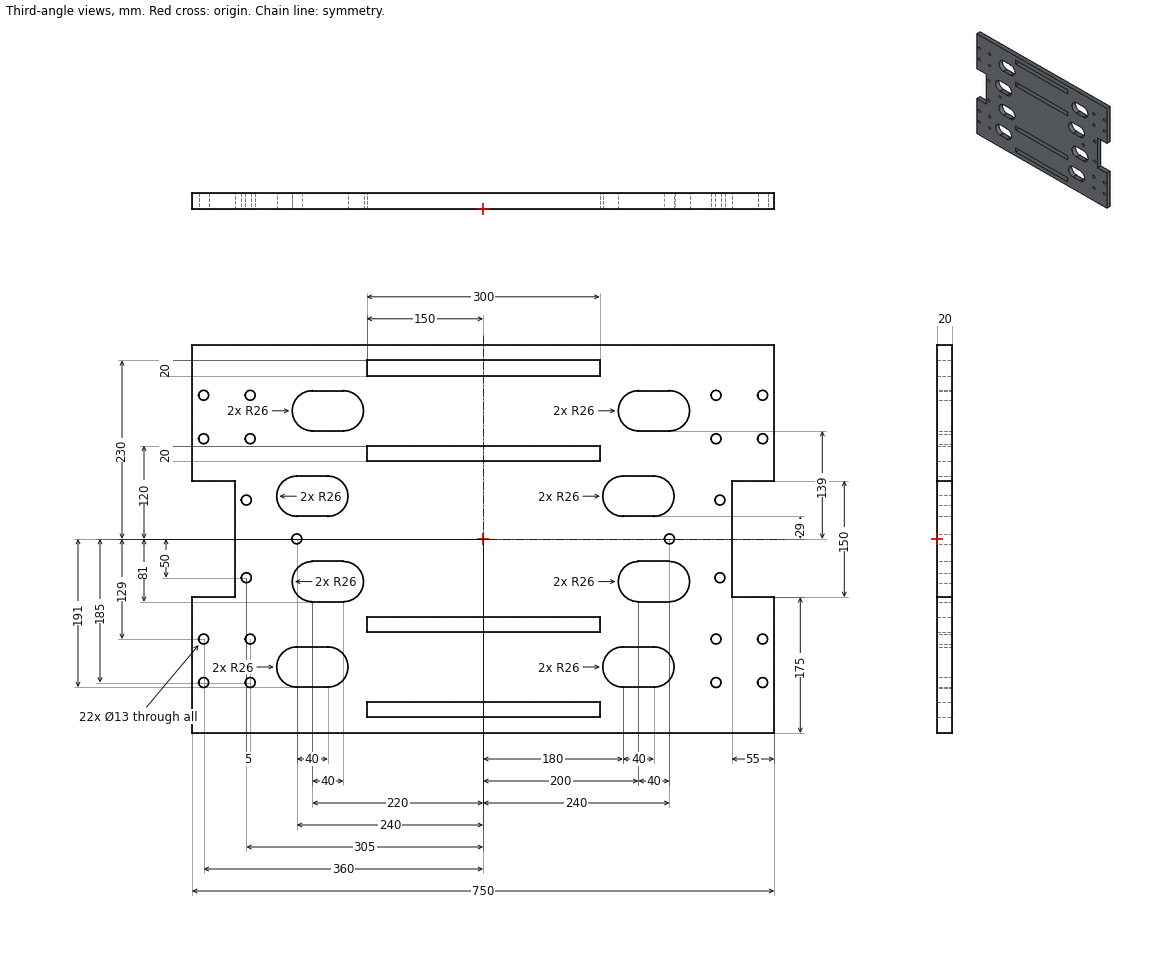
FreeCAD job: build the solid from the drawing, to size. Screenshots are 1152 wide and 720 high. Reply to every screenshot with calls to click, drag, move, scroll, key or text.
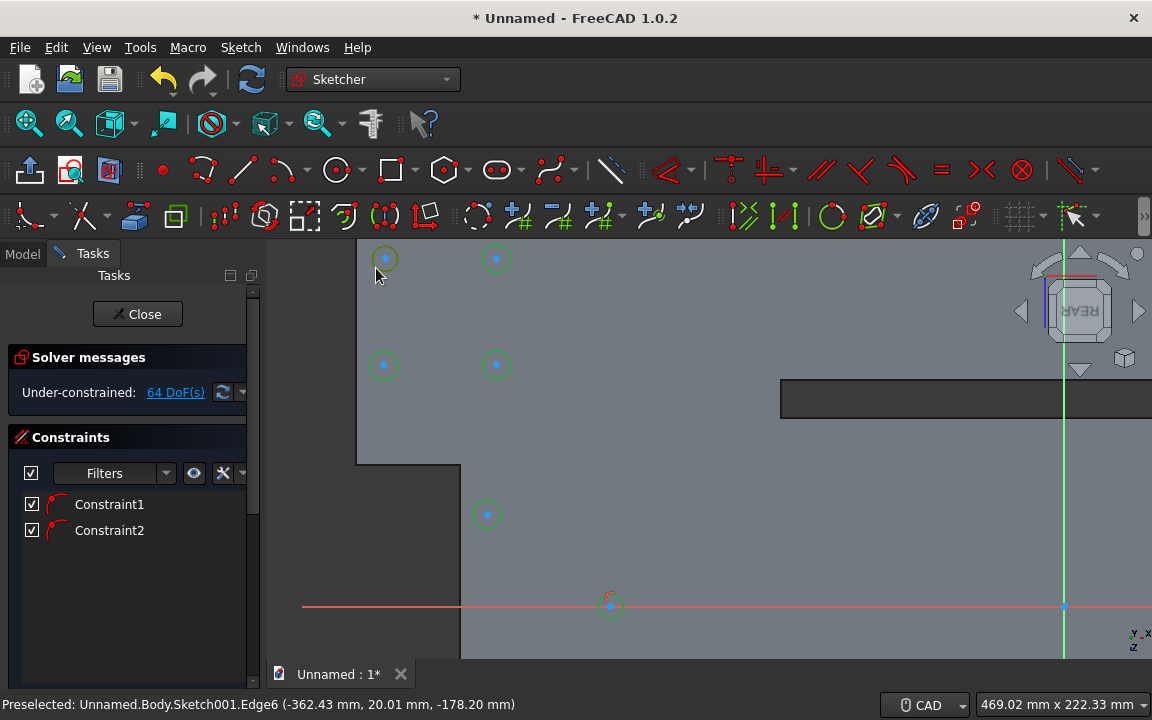
scroll(394, 357, down, 5)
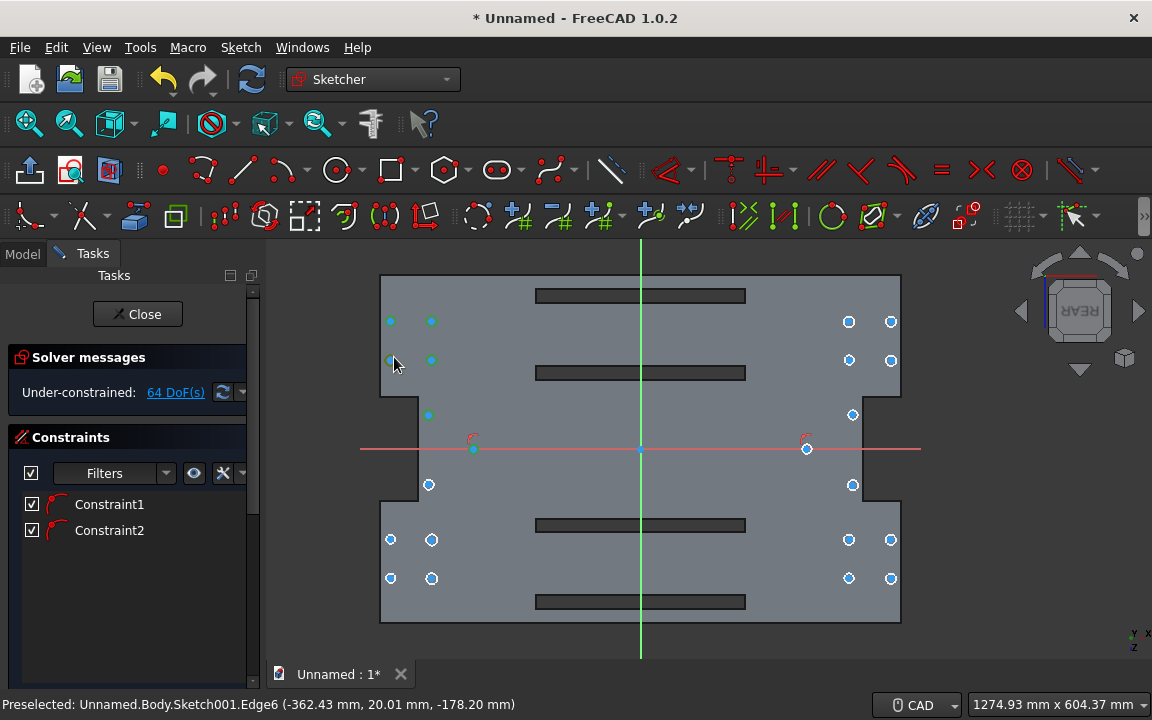
scroll(394, 536, up, 6)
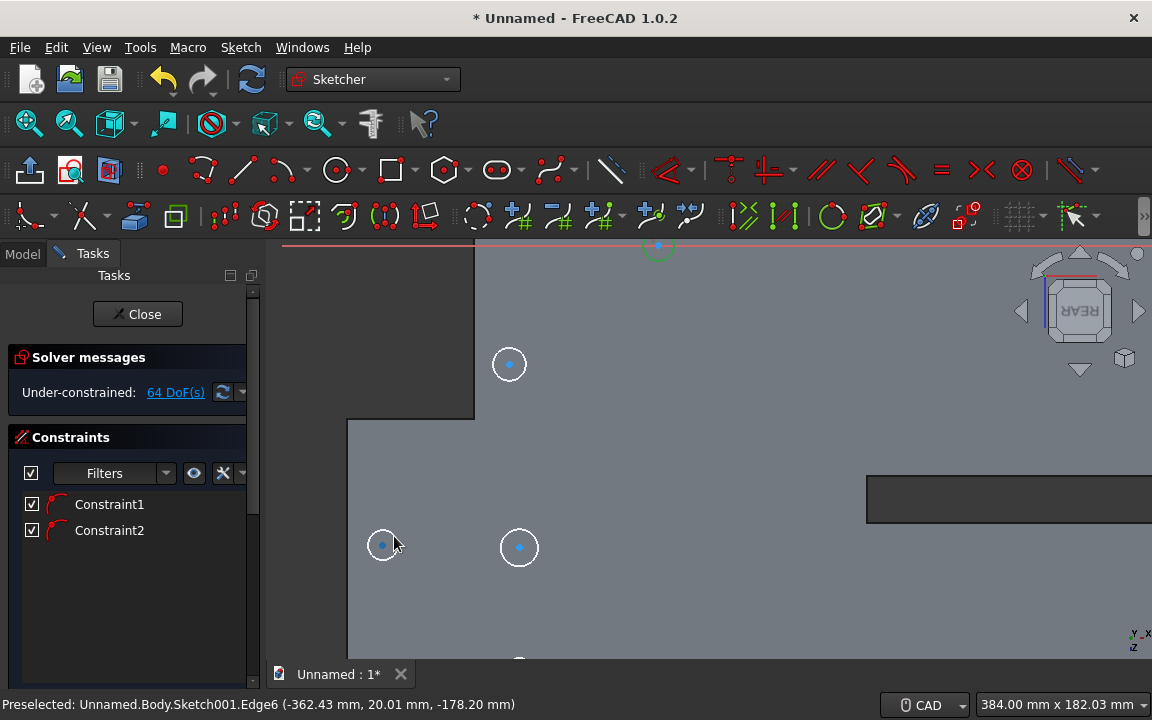
click(394, 534)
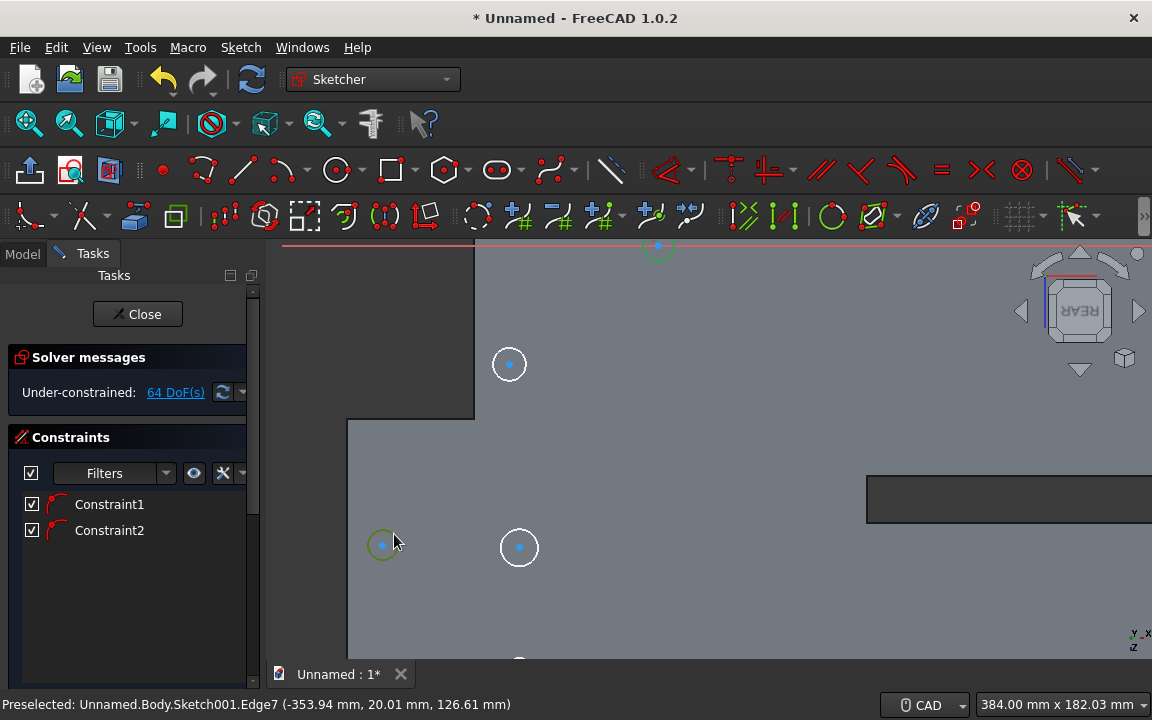
scroll(394, 537, down, 6)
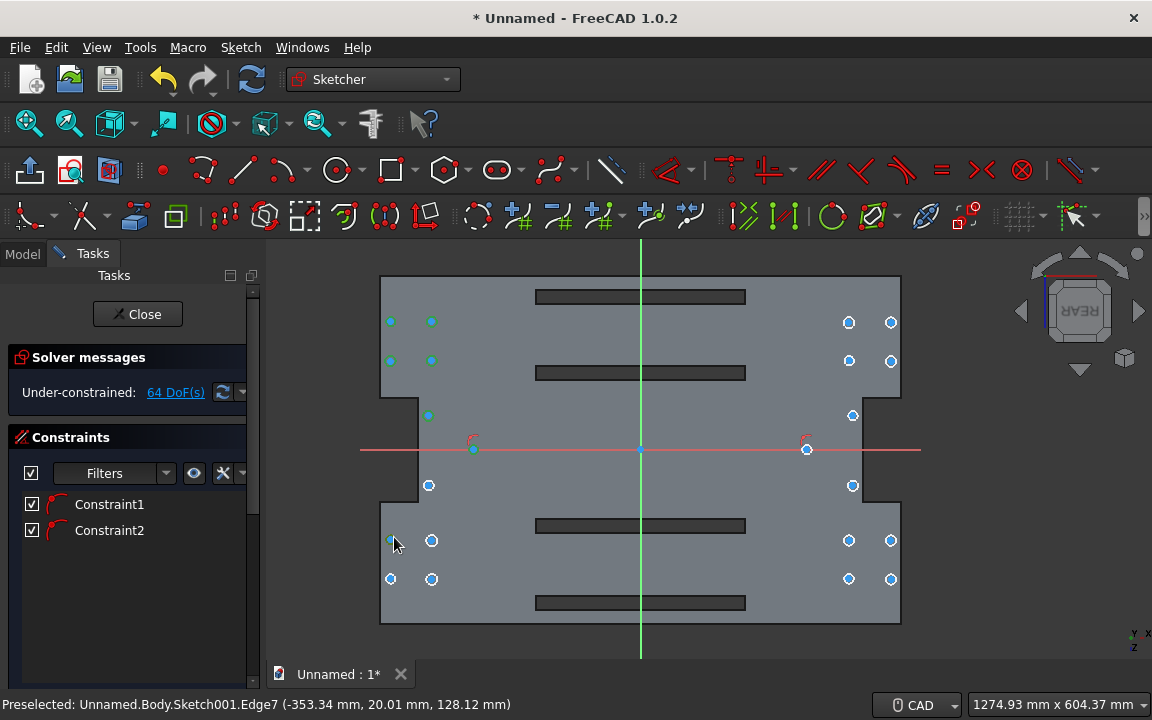
scroll(394, 576, up, 6)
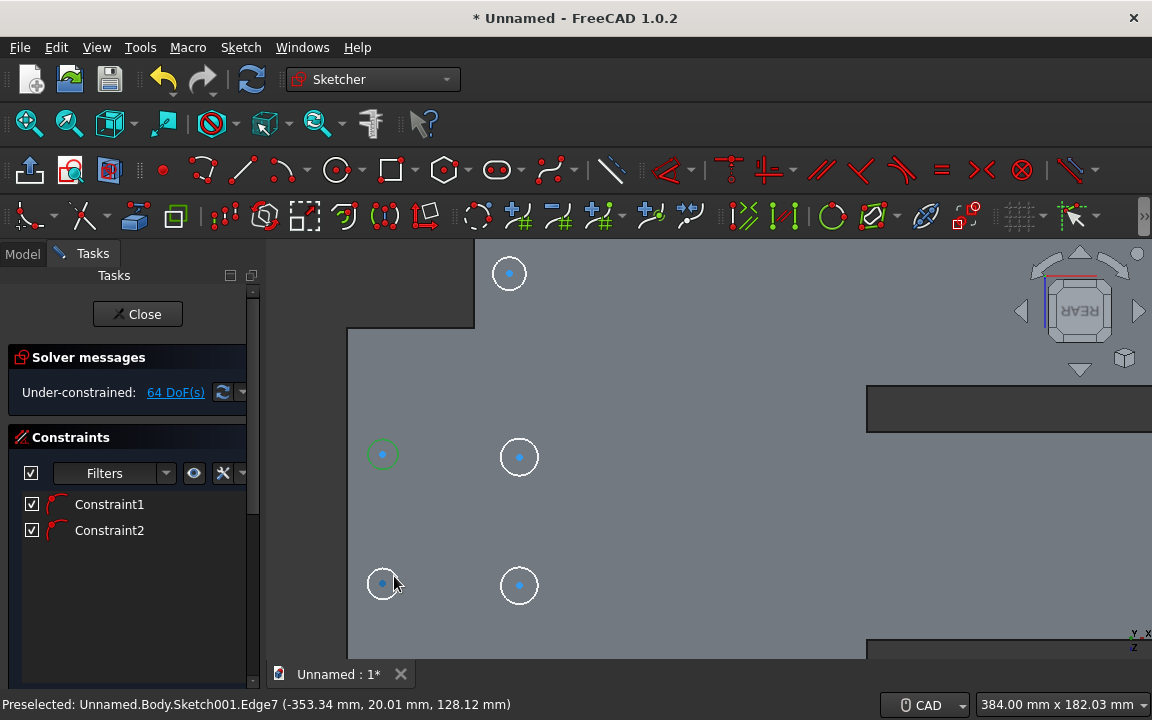
click(394, 573)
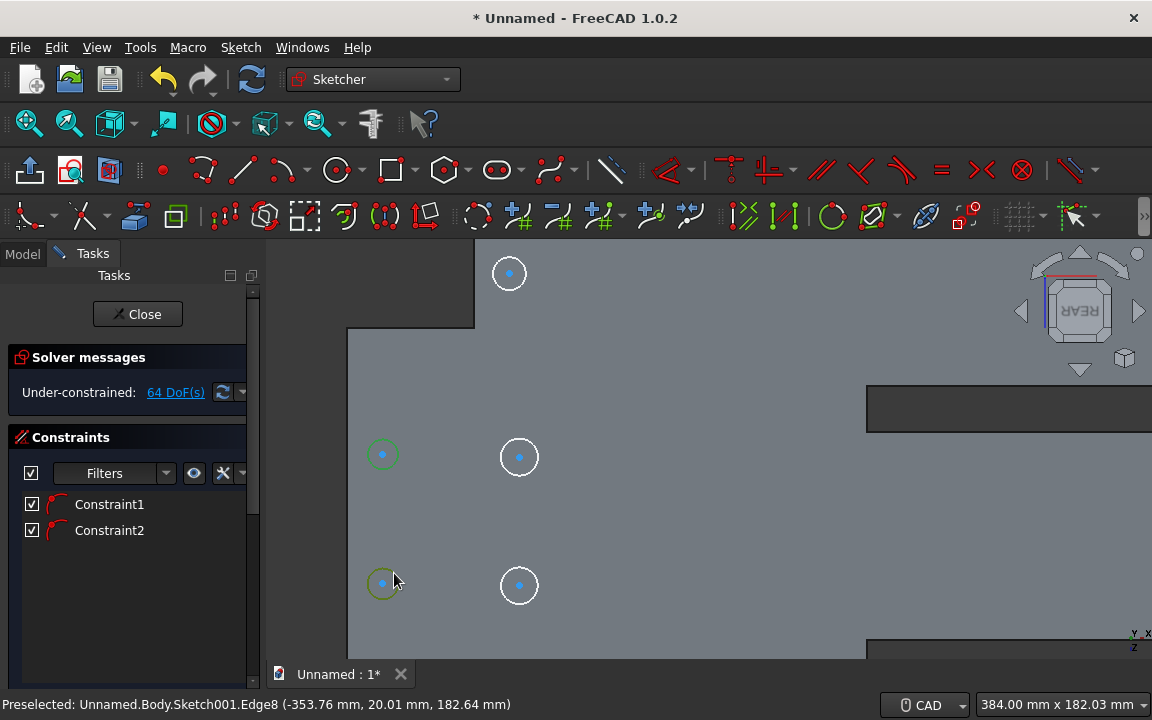
click(532, 444)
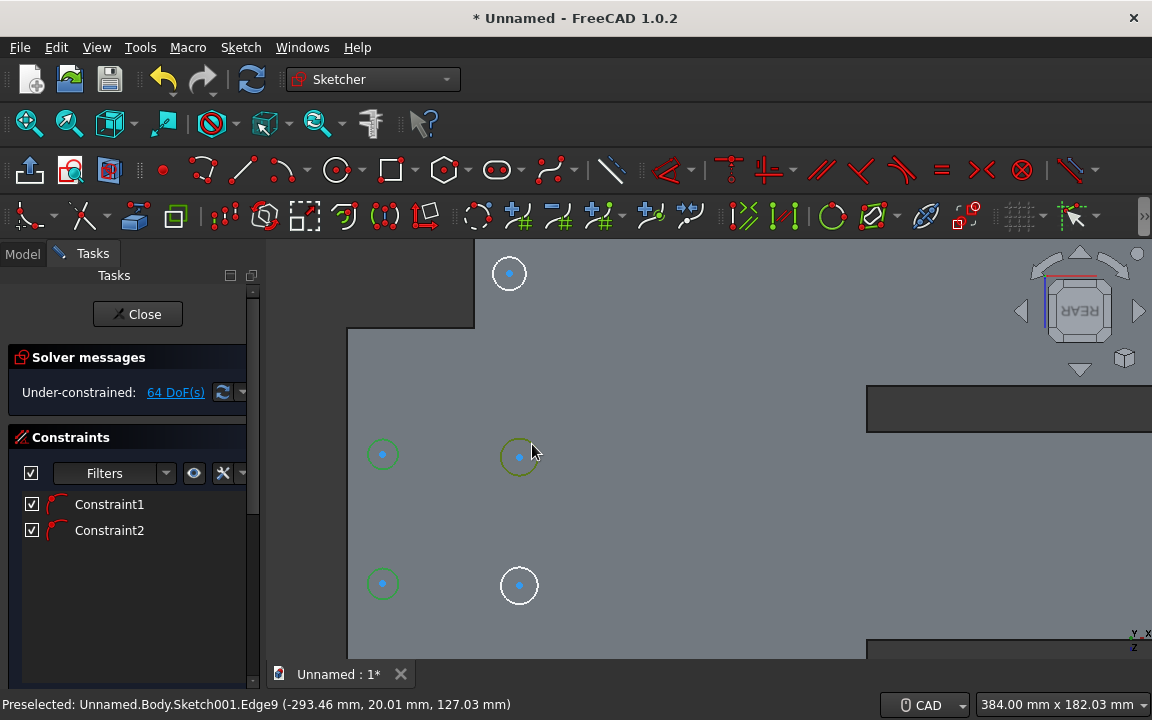
click(532, 573)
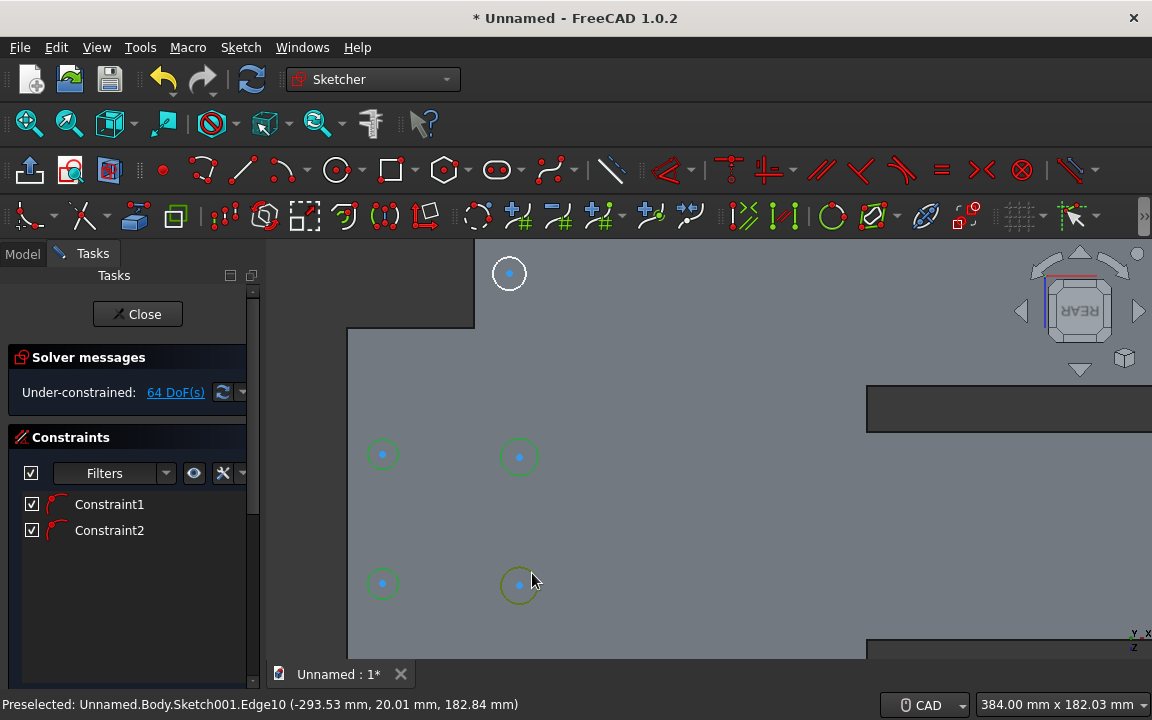
click(498, 285)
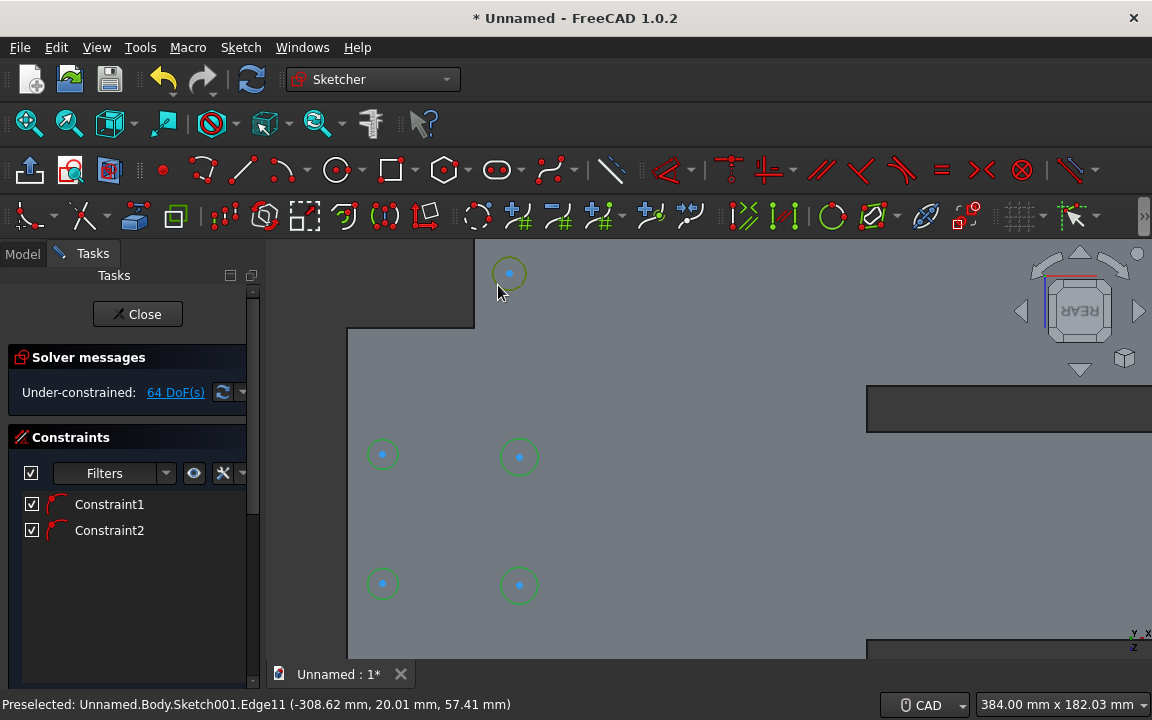
scroll(394, 576, down, 6)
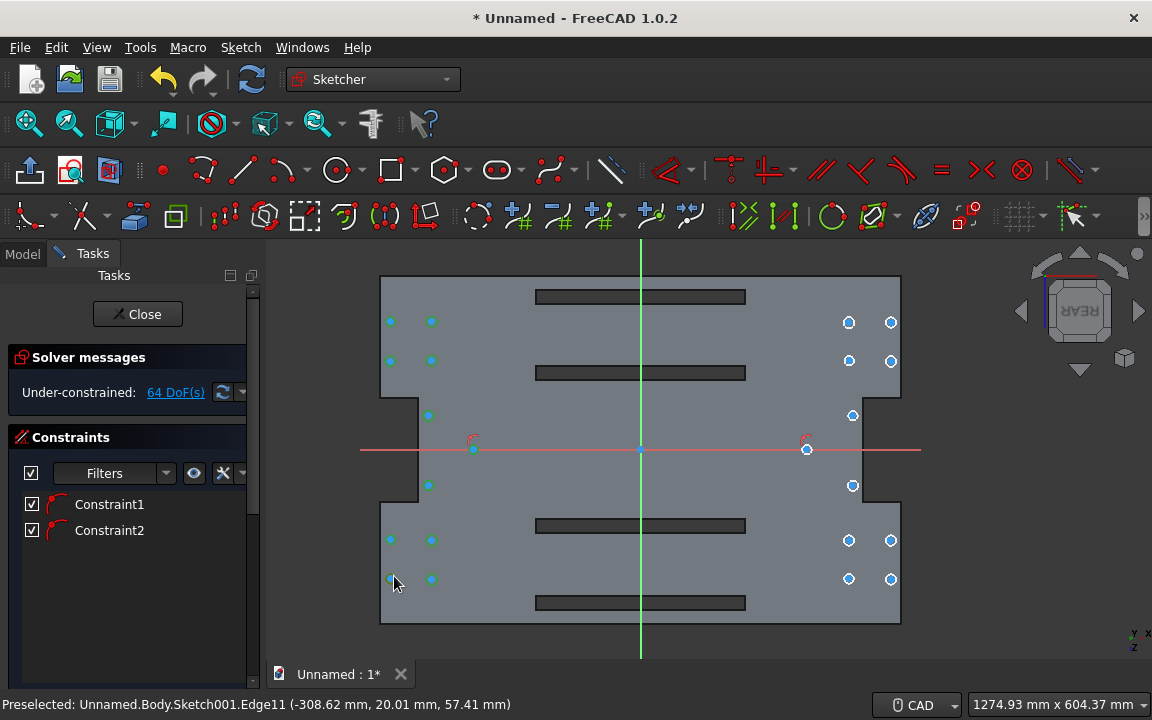
scroll(894, 537, up, 5)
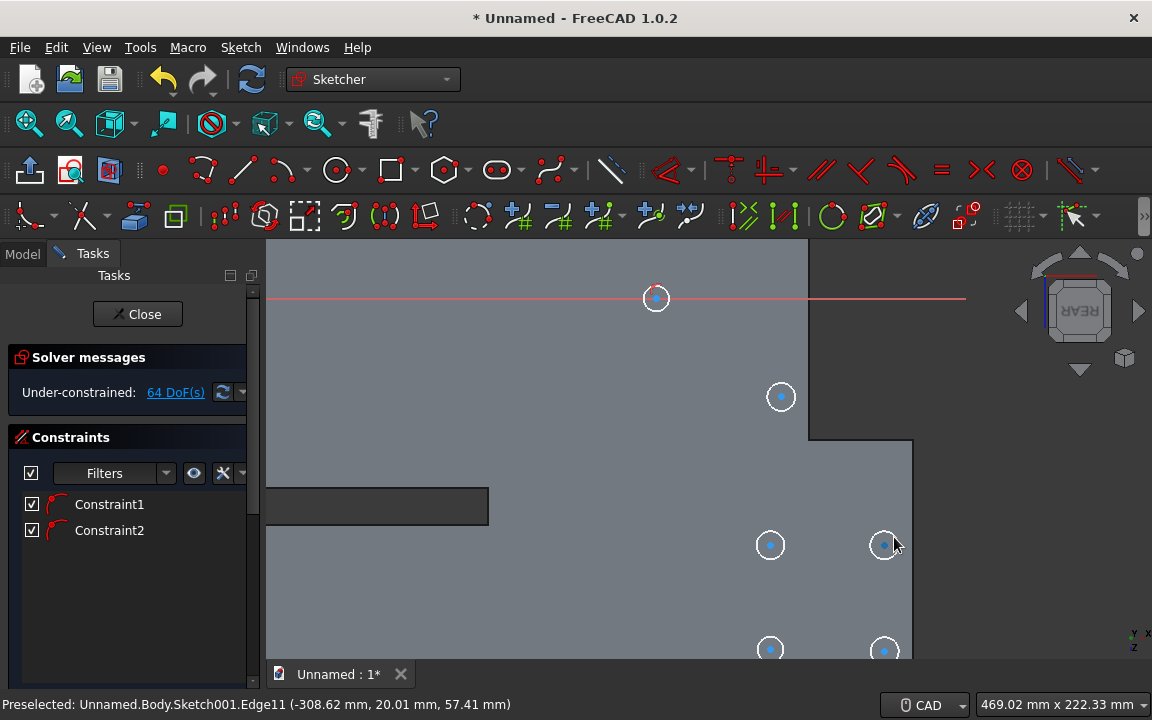
click(894, 535)